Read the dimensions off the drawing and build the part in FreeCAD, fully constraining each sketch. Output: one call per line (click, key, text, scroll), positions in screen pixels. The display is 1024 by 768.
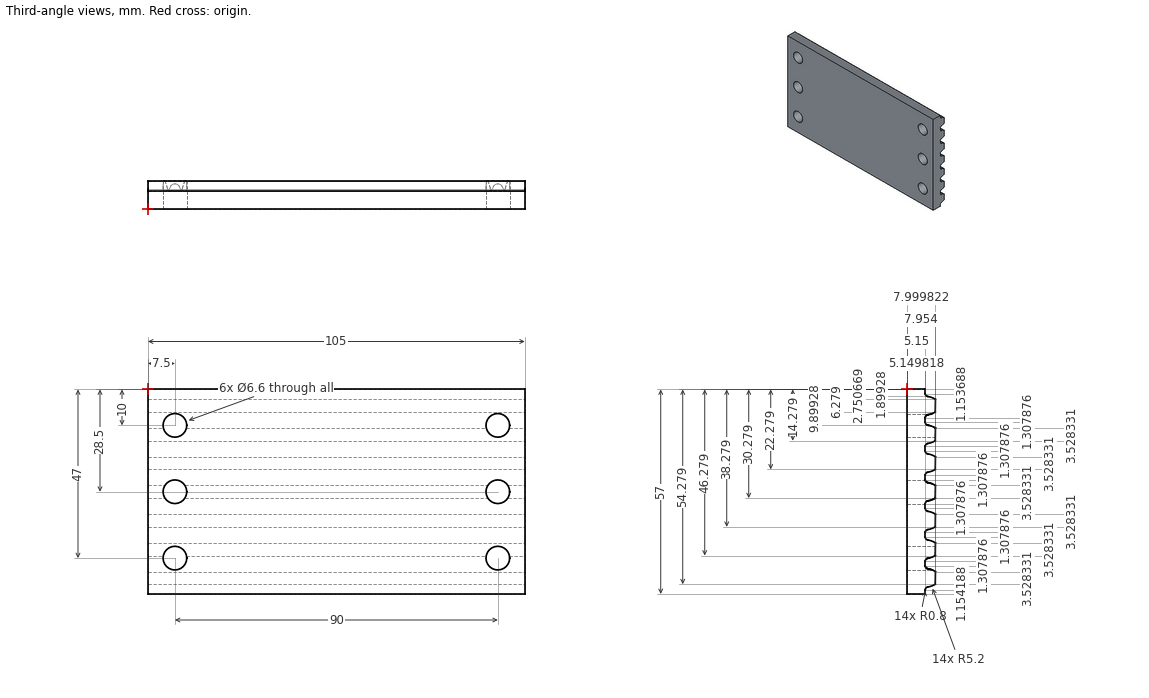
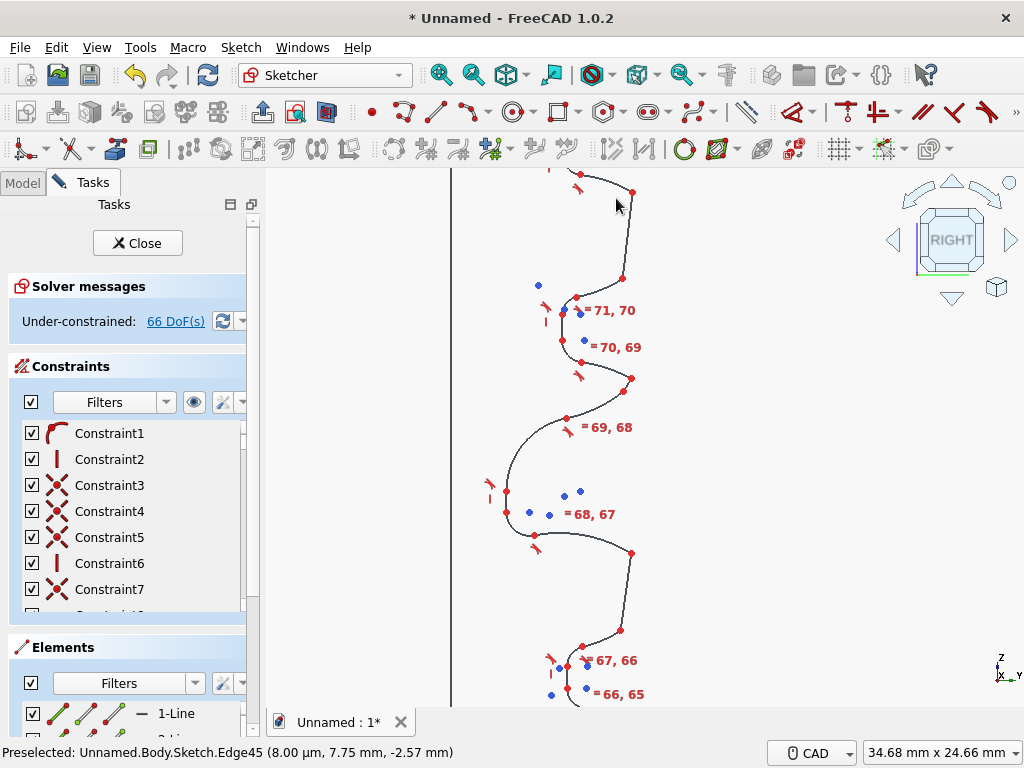
scroll(593, 296, down, 6)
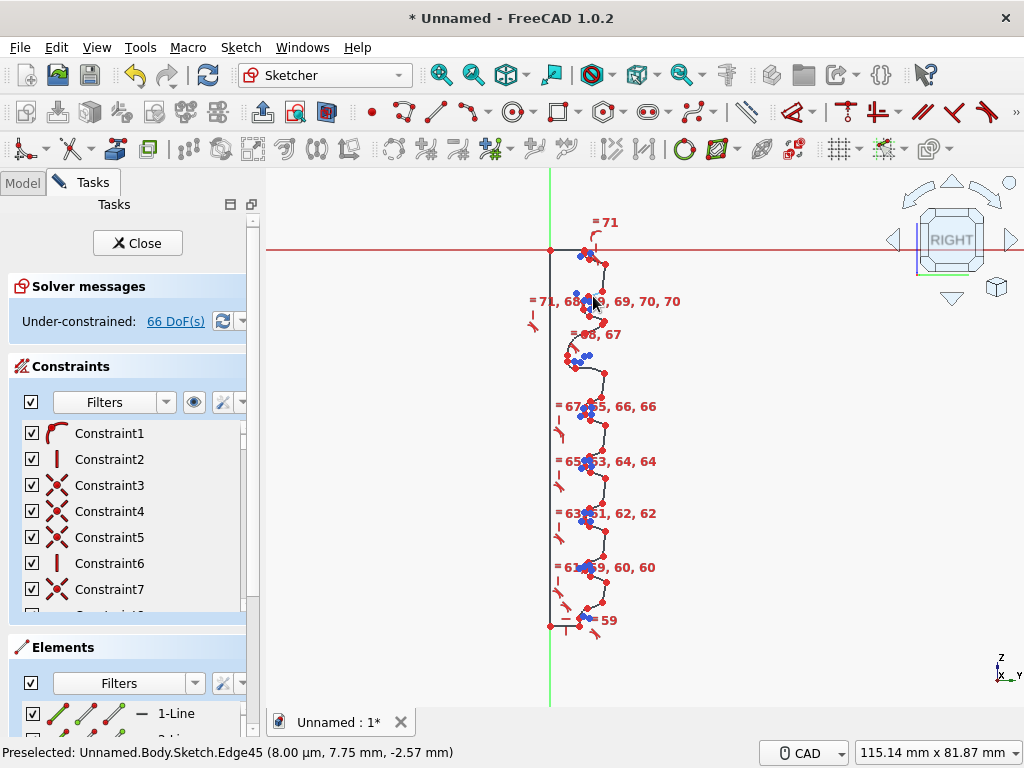
scroll(584, 610, up, 6)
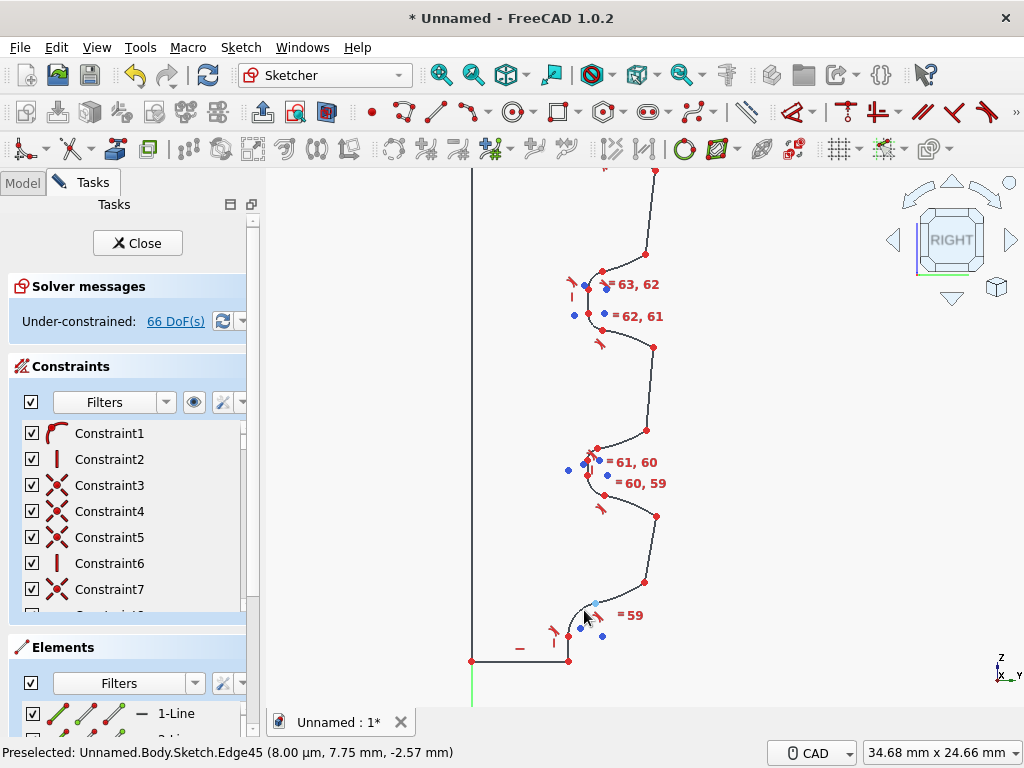
click(583, 609)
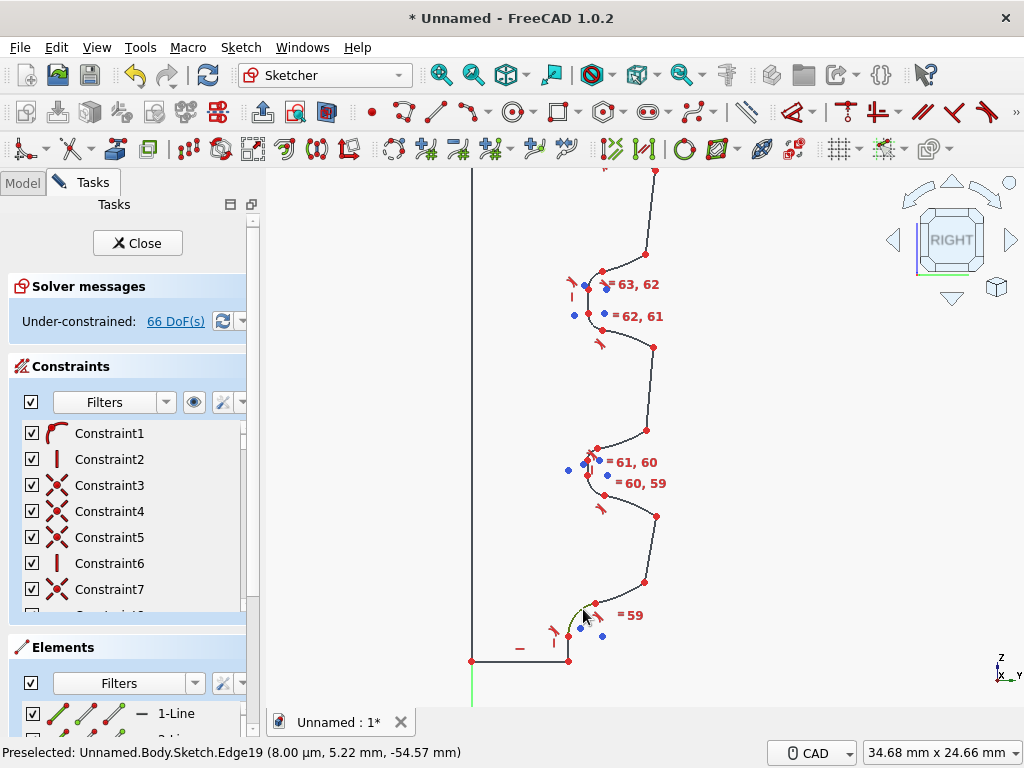
scroll(590, 453, up, 3)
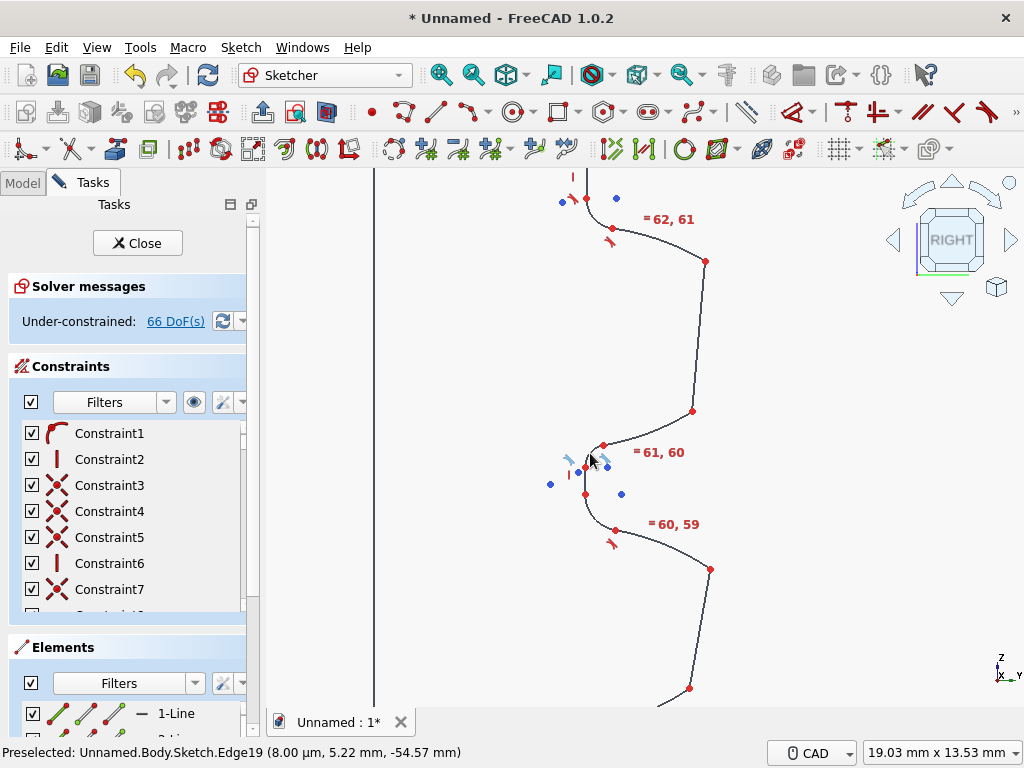
click(590, 453)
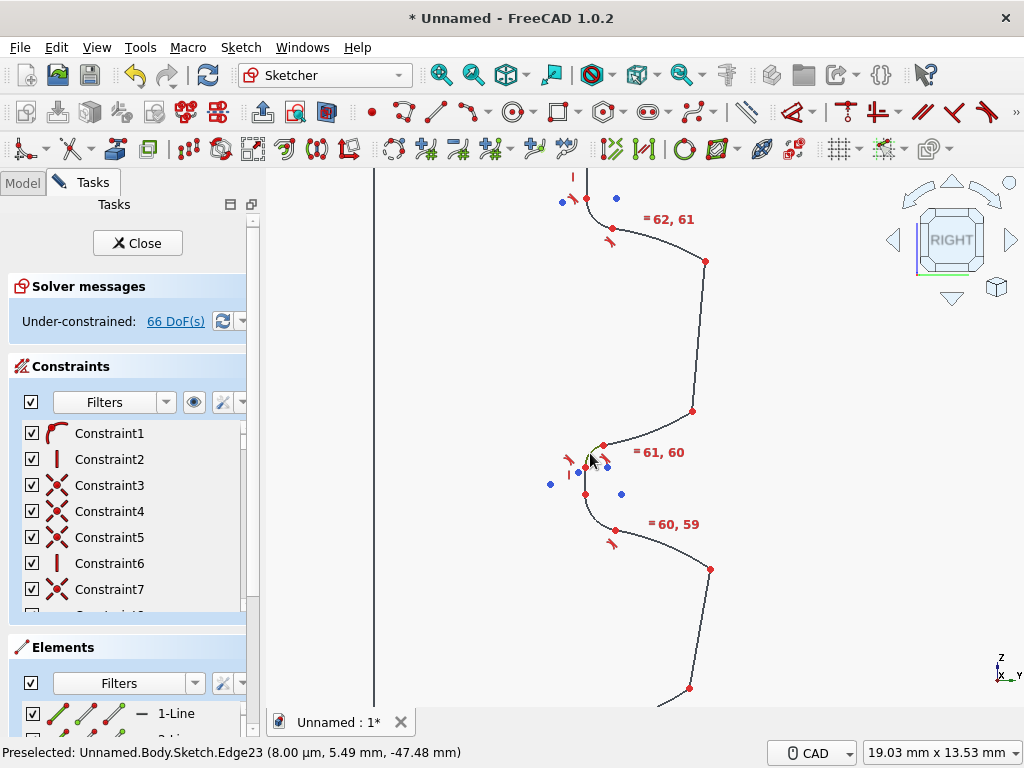
scroll(585, 585, down, 9)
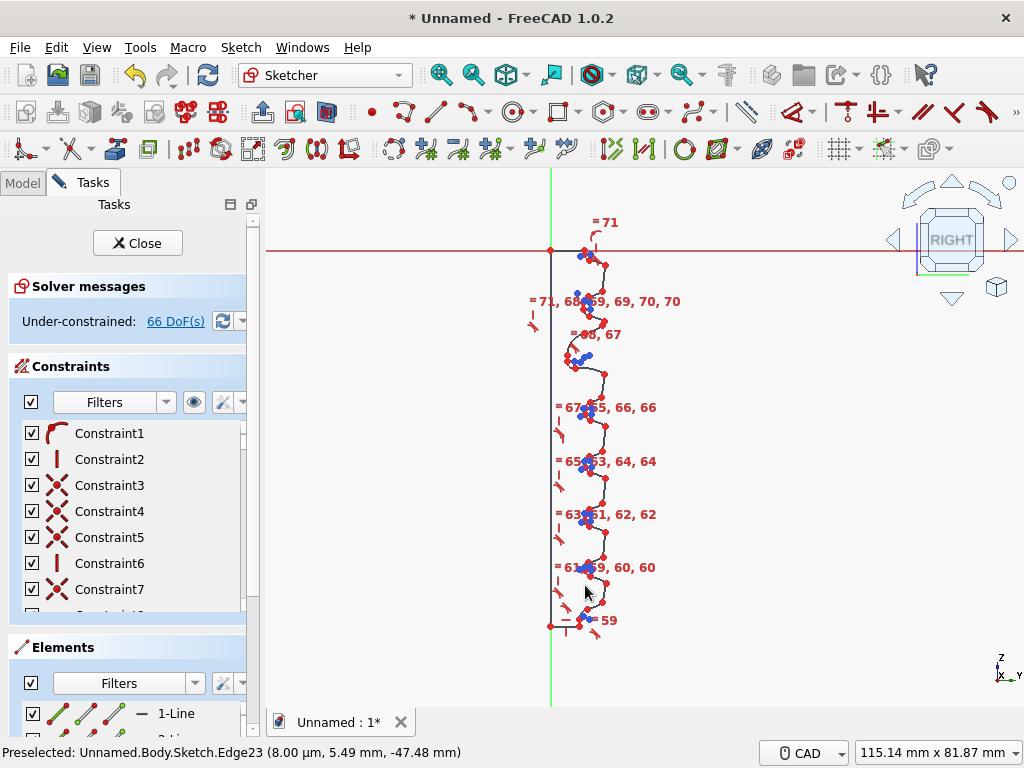
scroll(588, 510, up, 10)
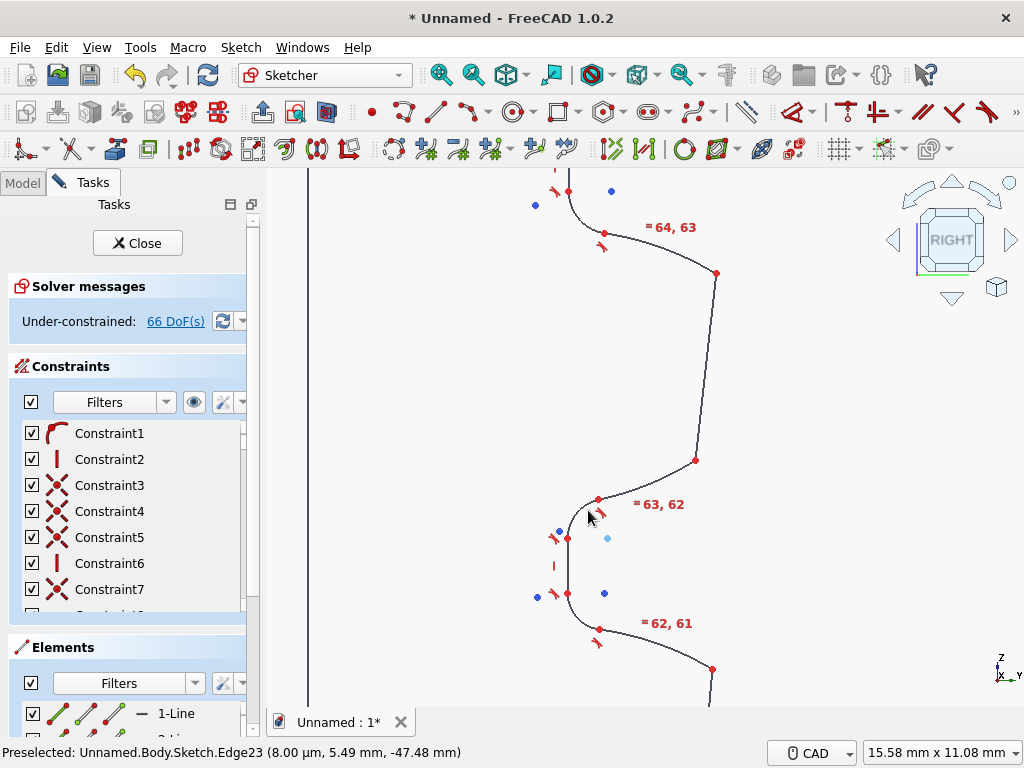
click(584, 506)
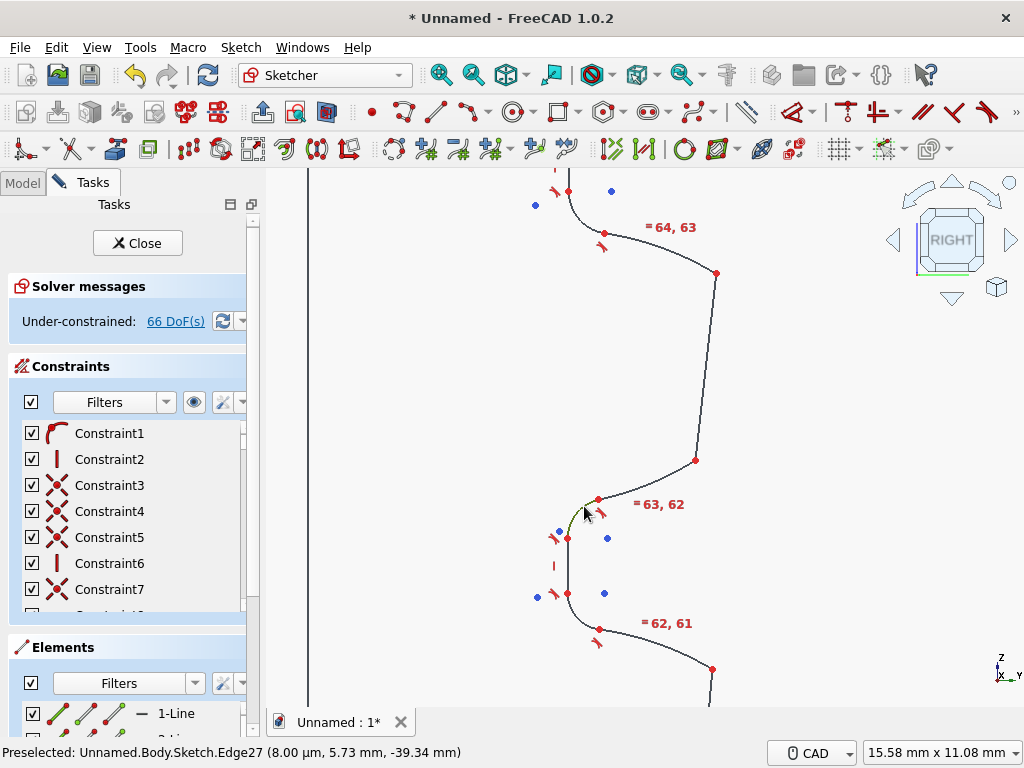
scroll(588, 510, down, 10)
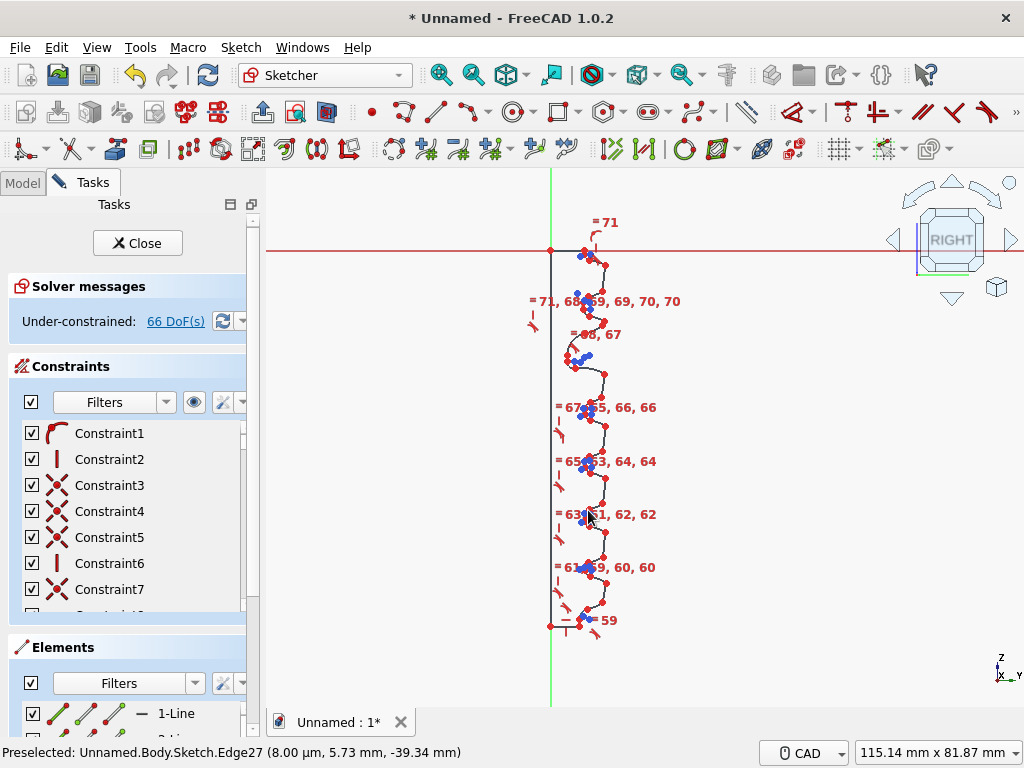
scroll(588, 457, up, 11)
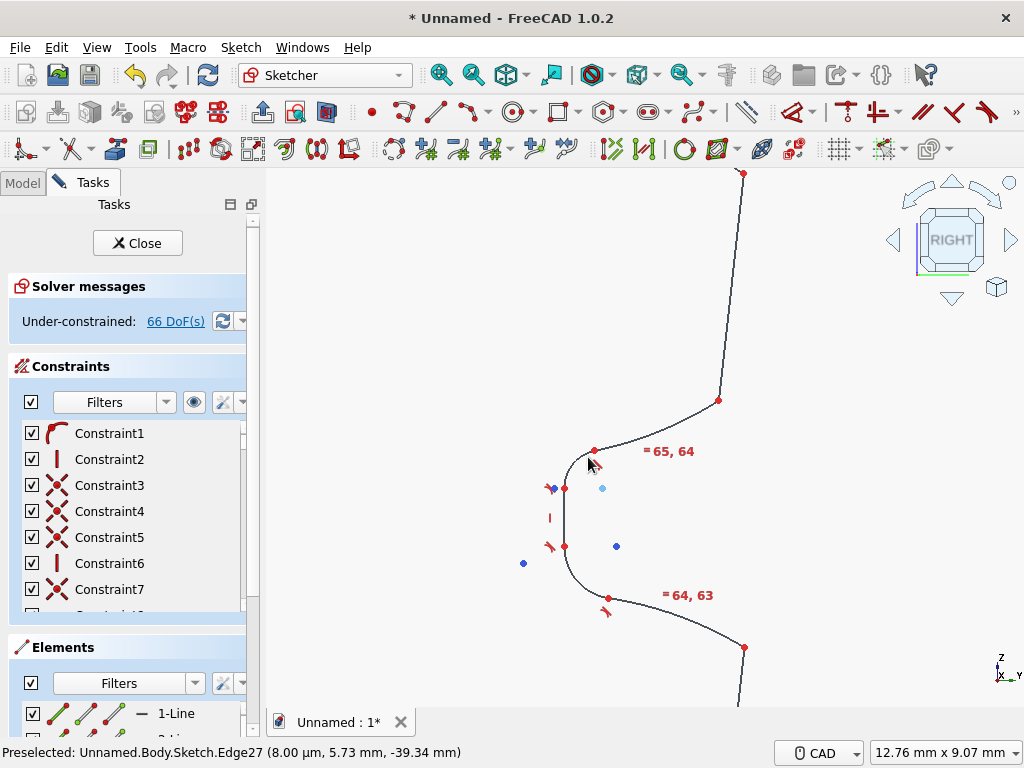
click(581, 457)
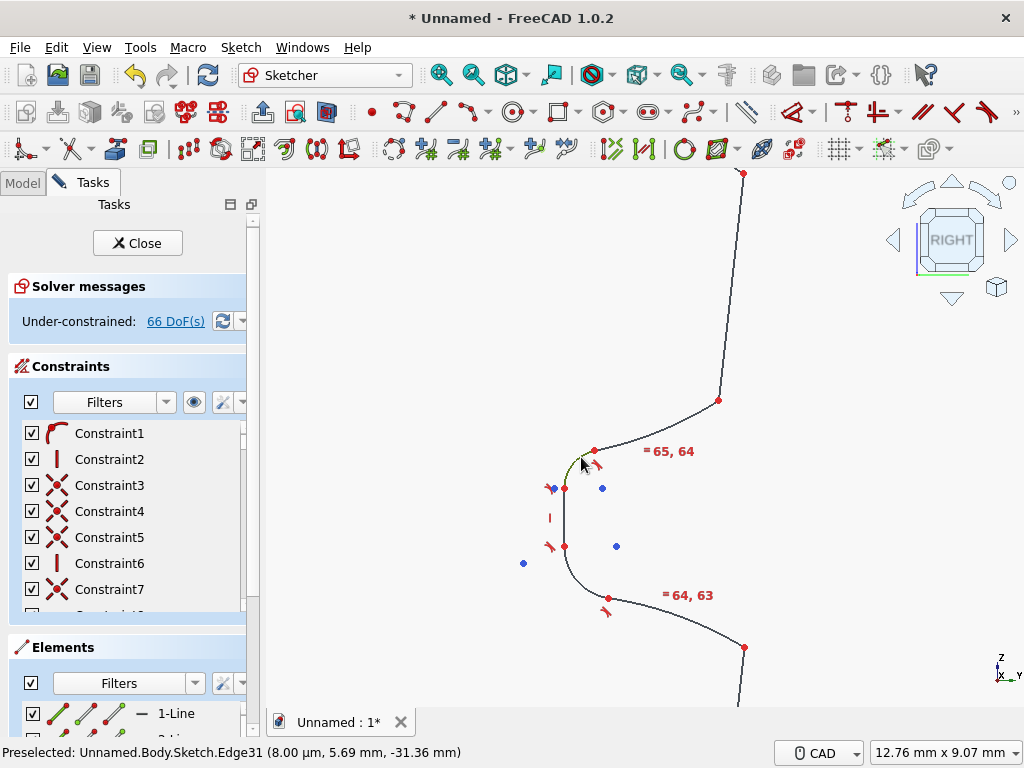
scroll(588, 456, down, 11)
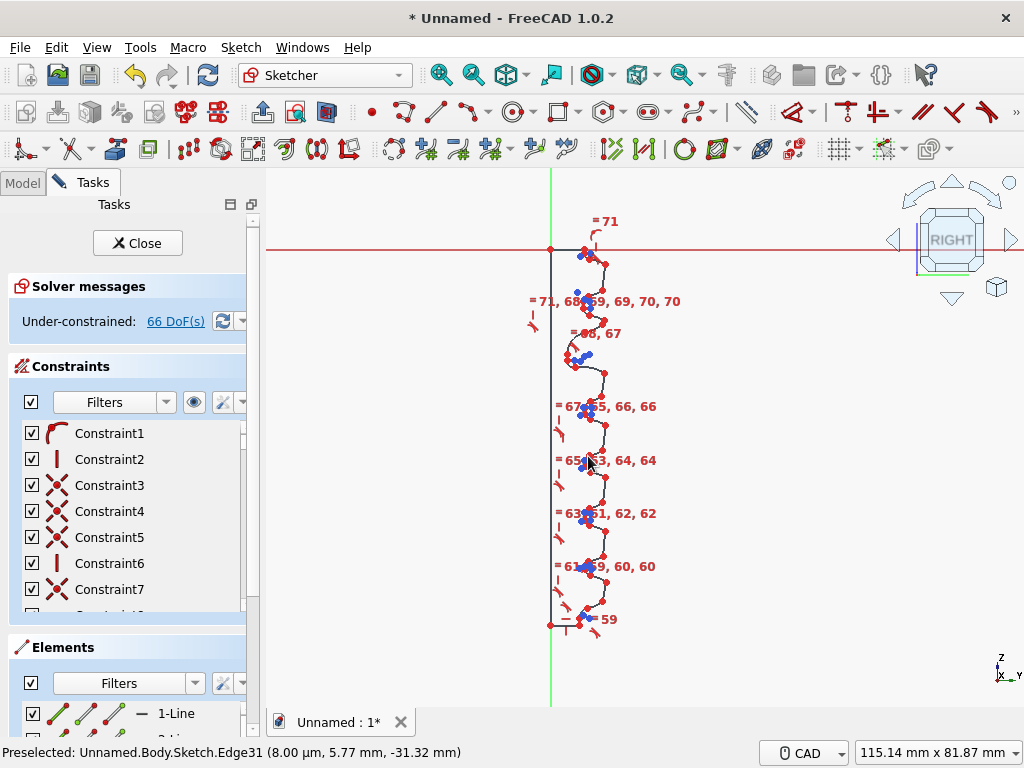
scroll(588, 402, up, 9)